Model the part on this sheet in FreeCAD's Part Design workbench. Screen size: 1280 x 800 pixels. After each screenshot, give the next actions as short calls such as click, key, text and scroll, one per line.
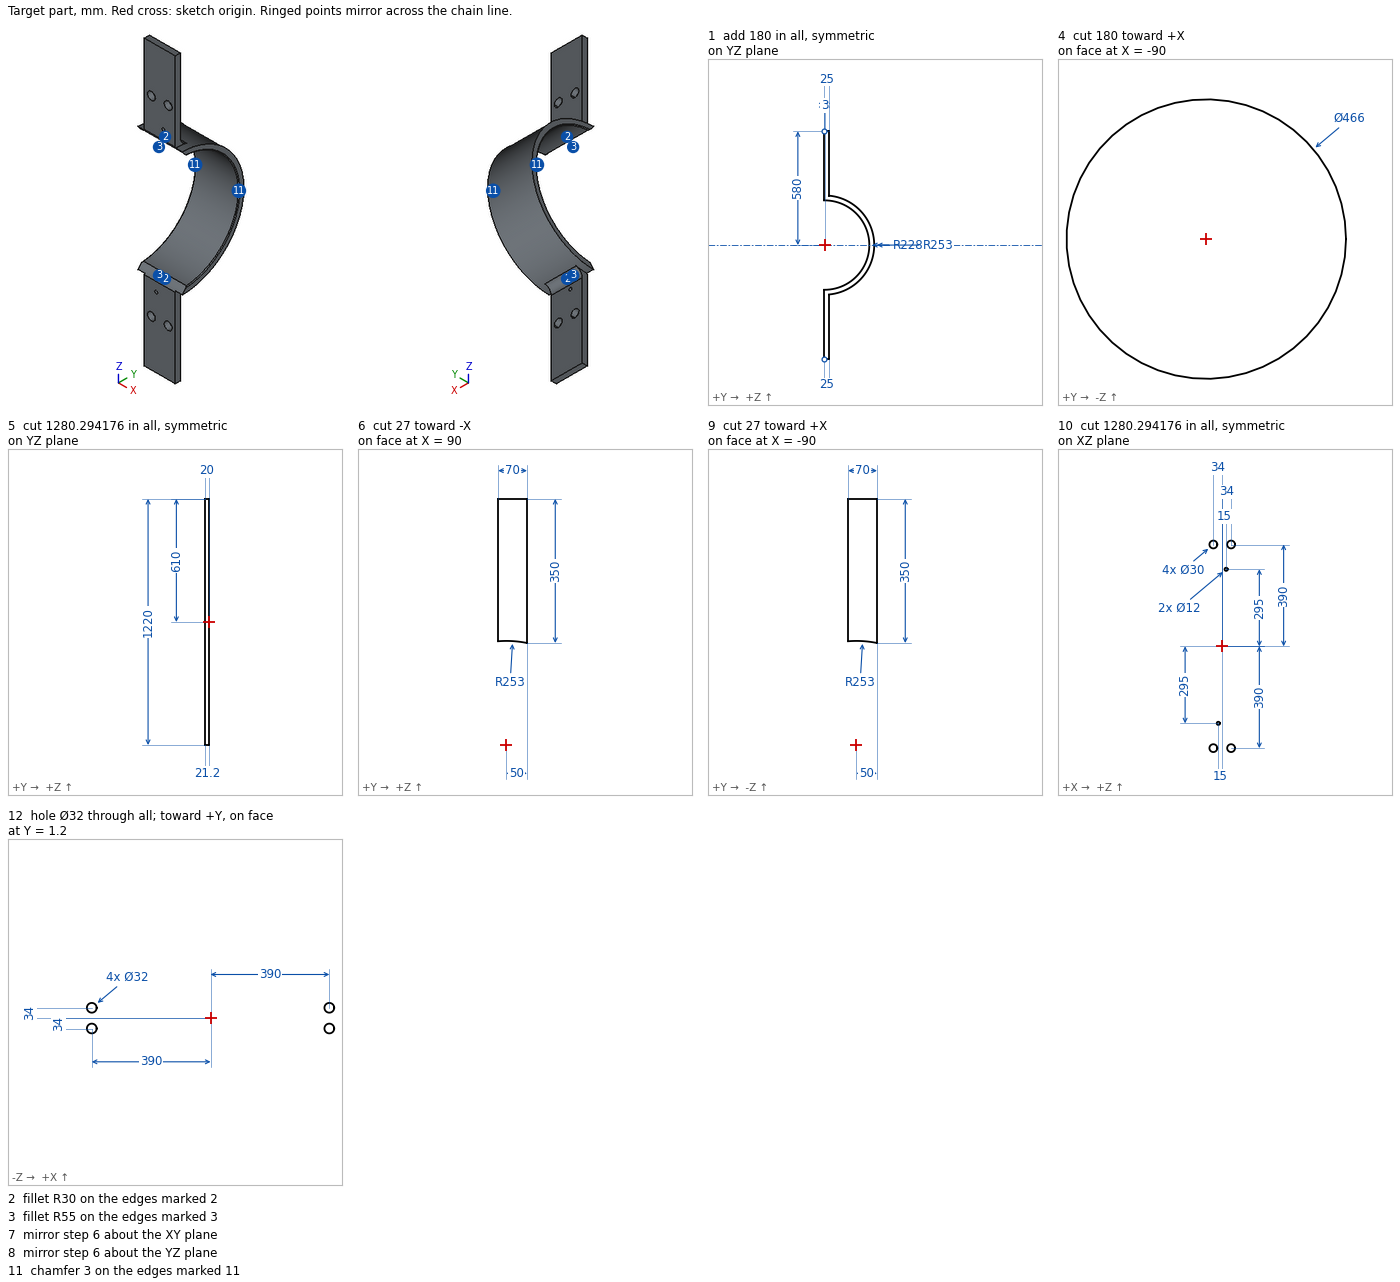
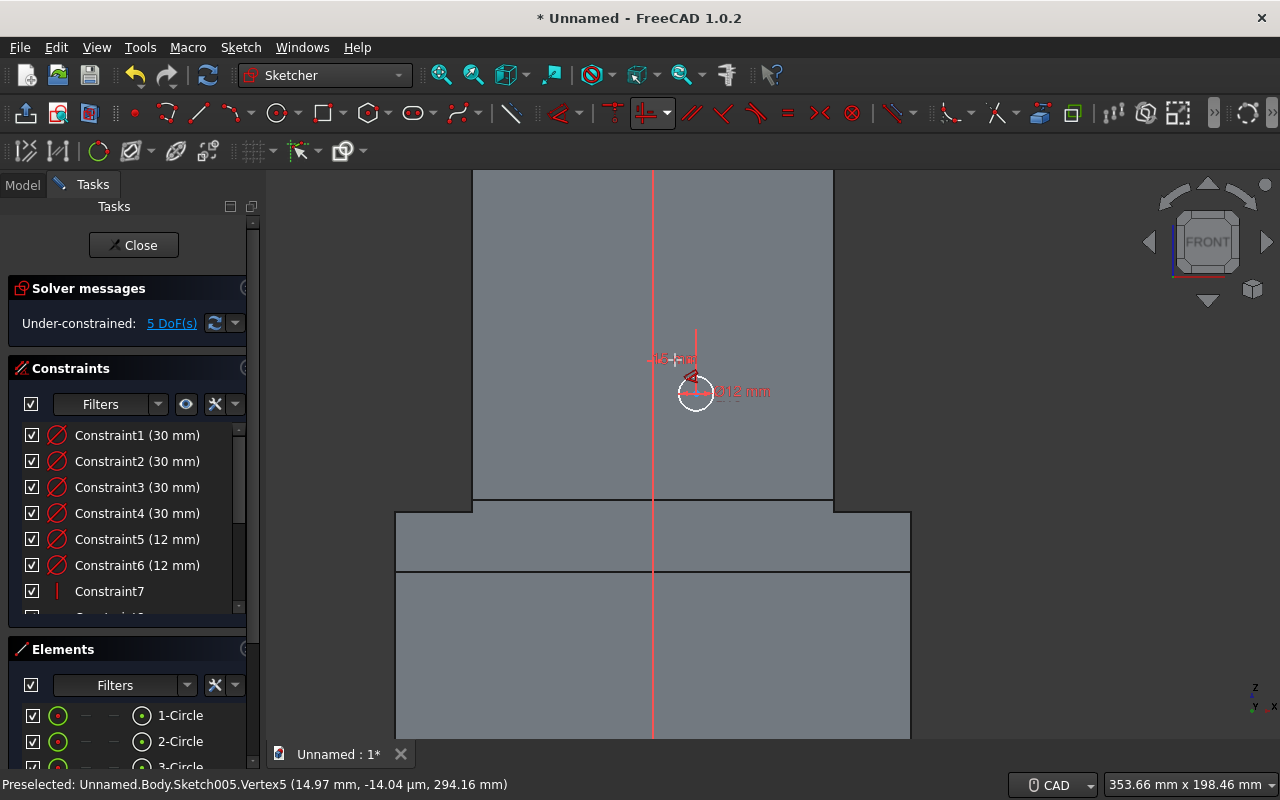
scroll(715, 300, down, 9)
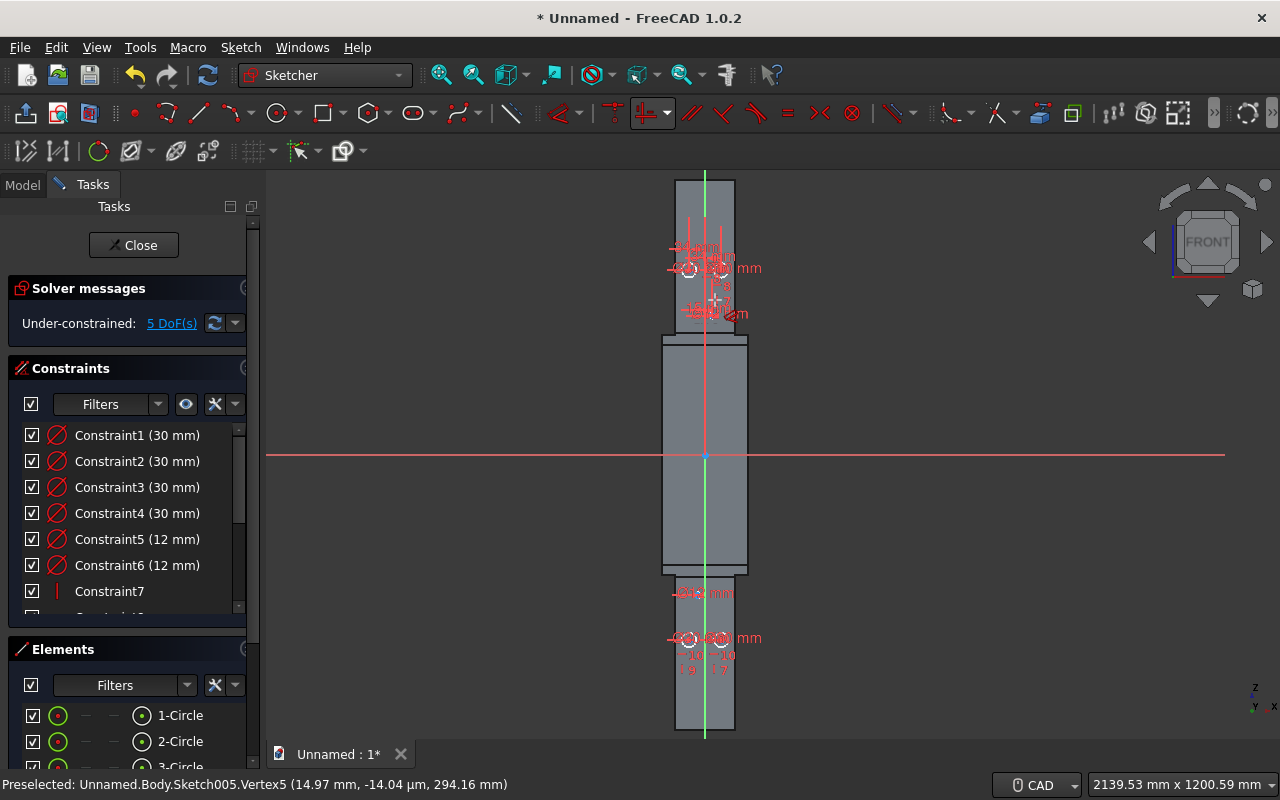
scroll(698, 595, up, 9)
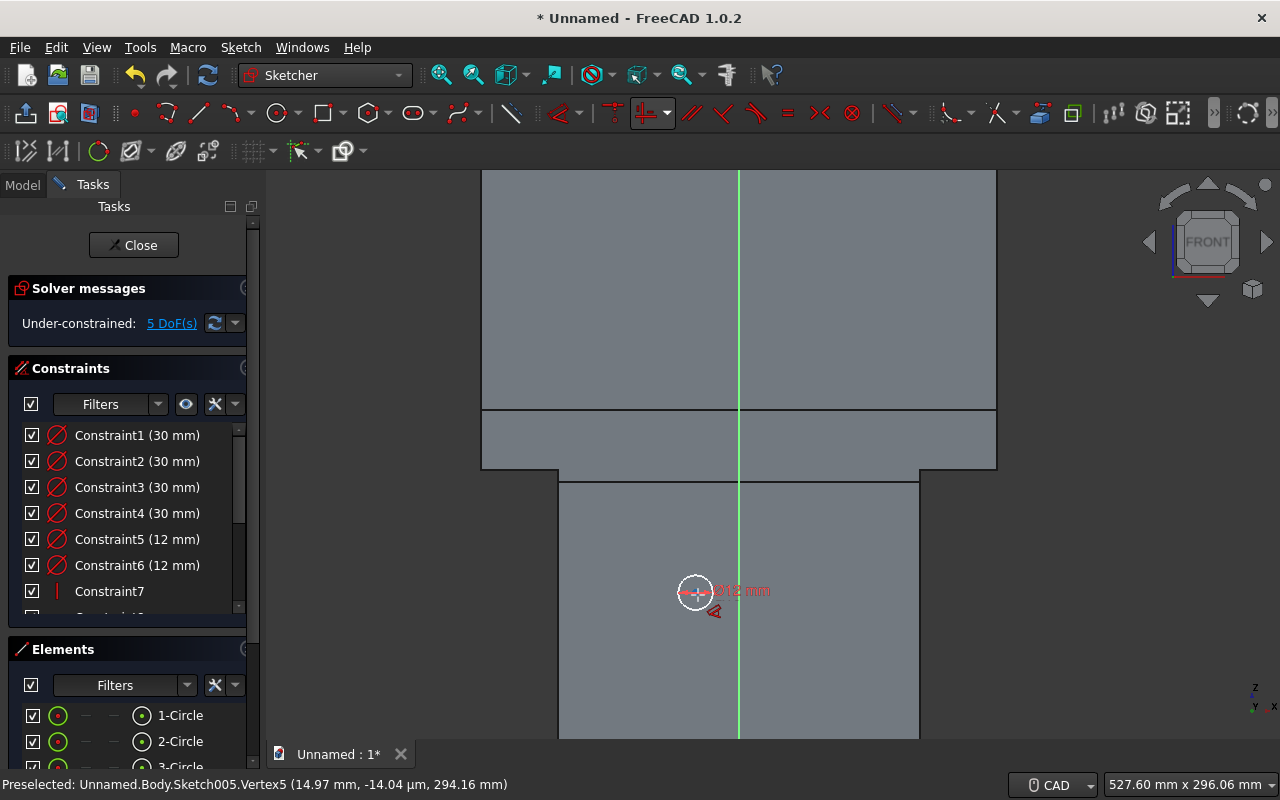
click(696, 593)
click(717, 627)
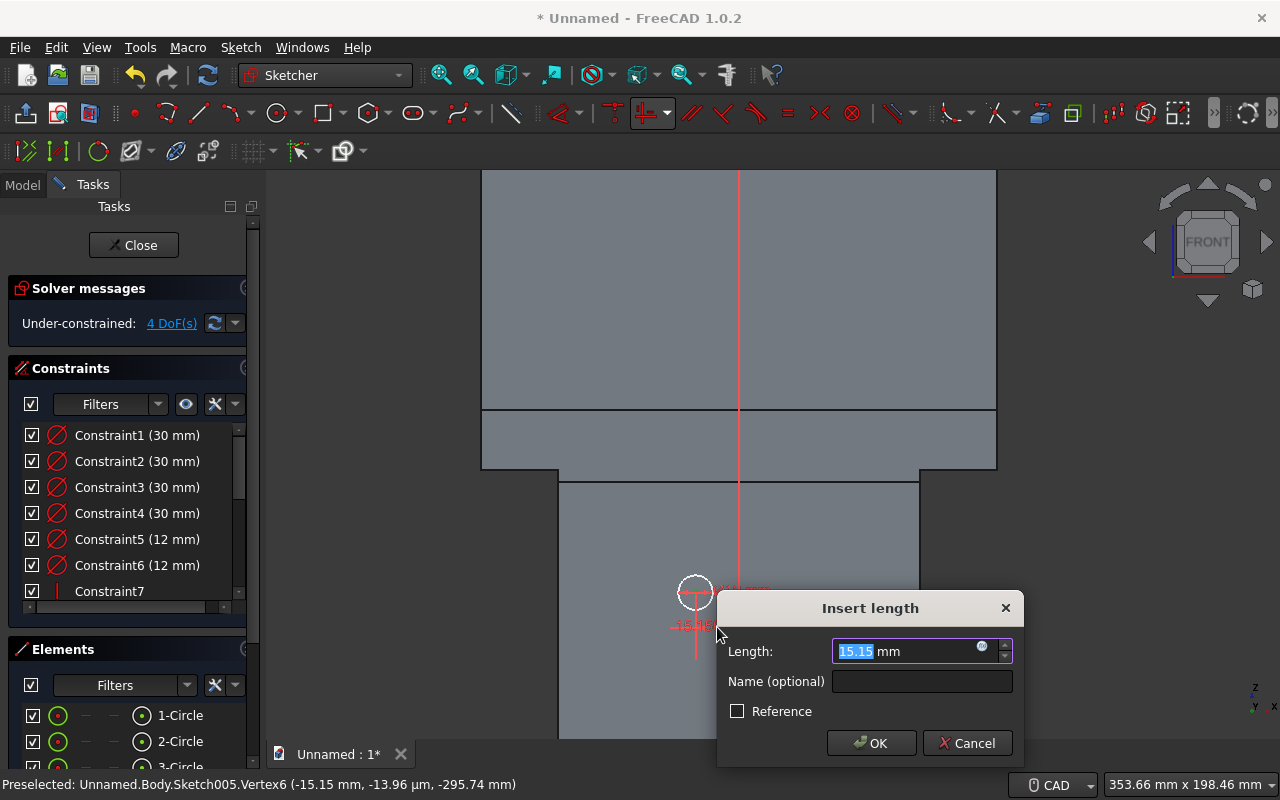
text(15)
key(Return)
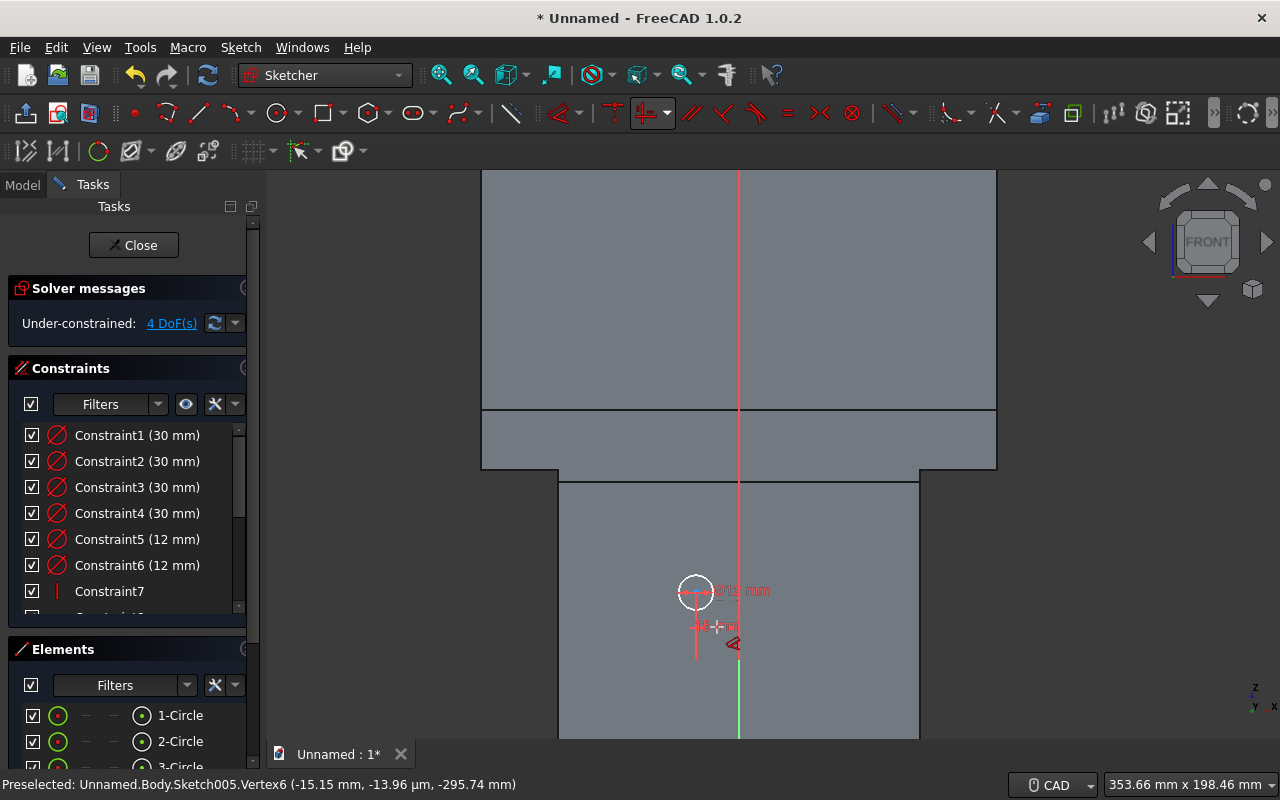
scroll(698, 595, down, 9)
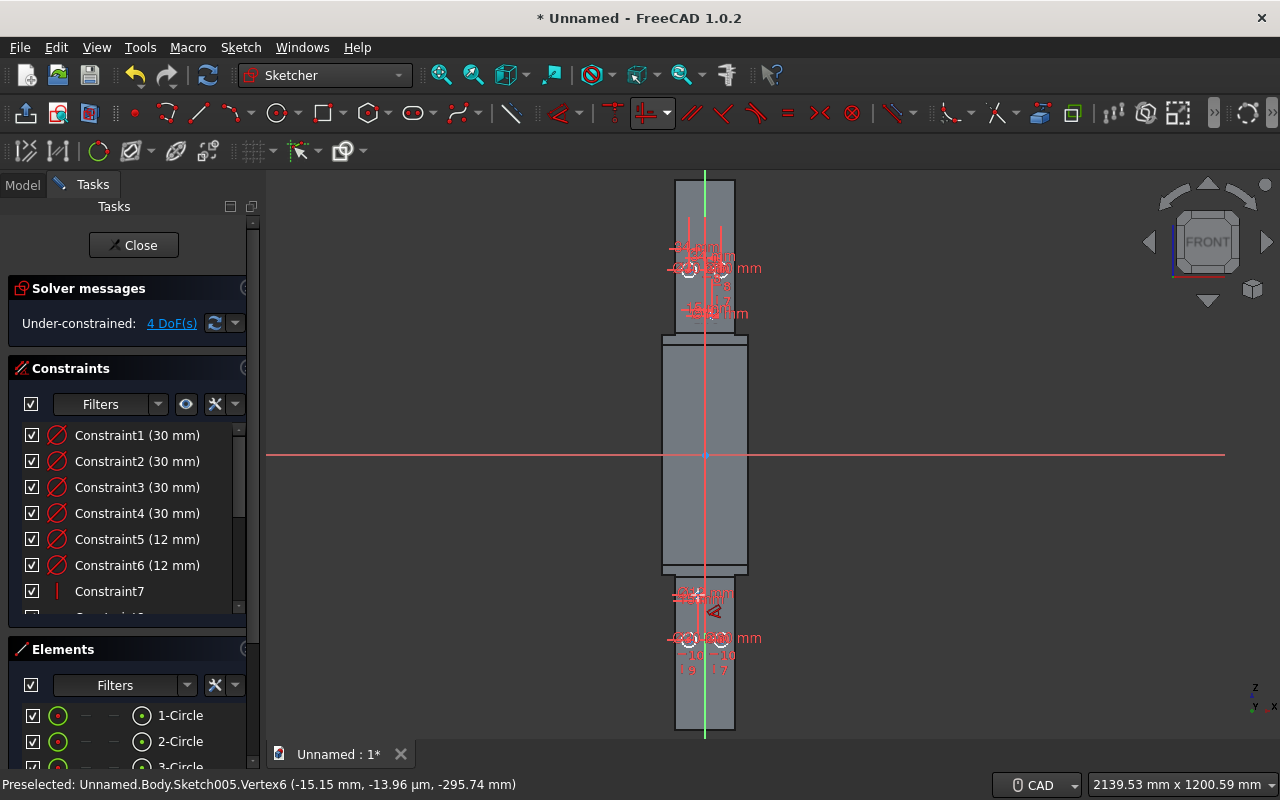
click(721, 270)
click(755, 363)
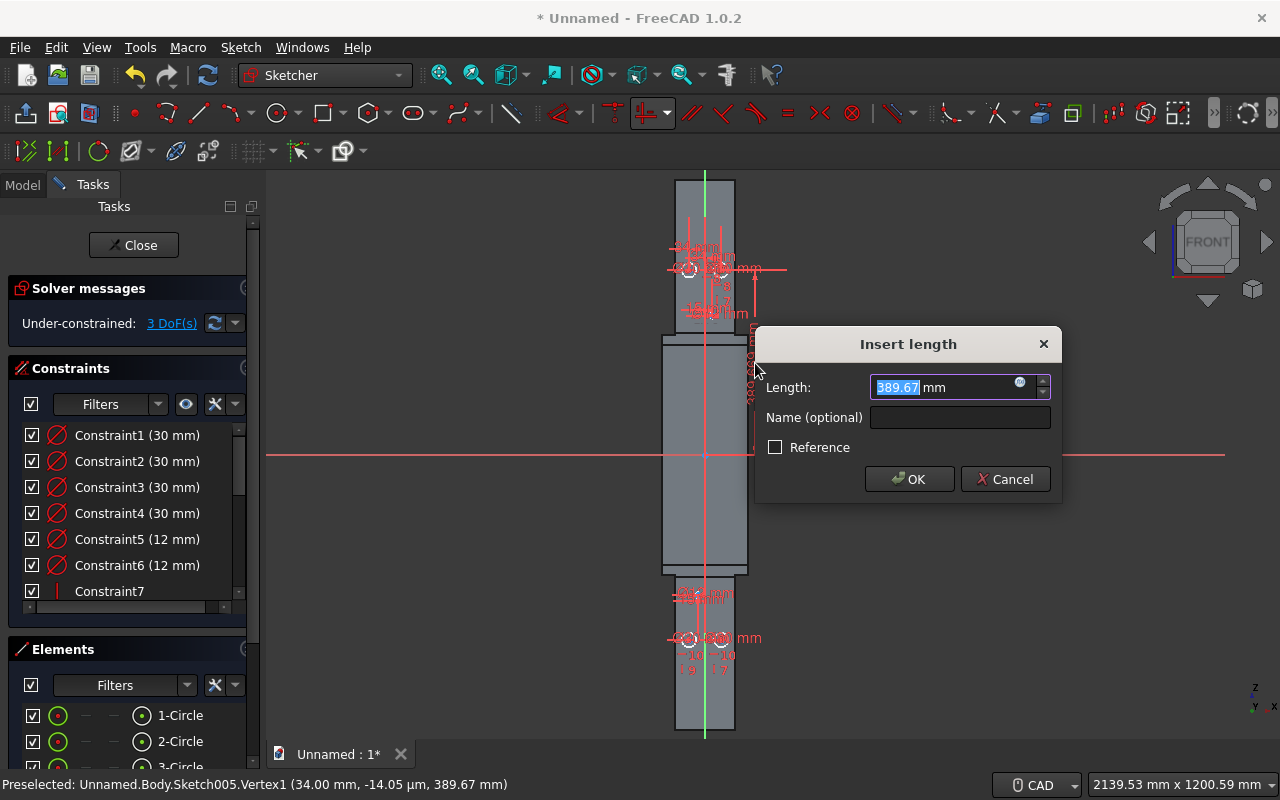
text(390)
key(Return)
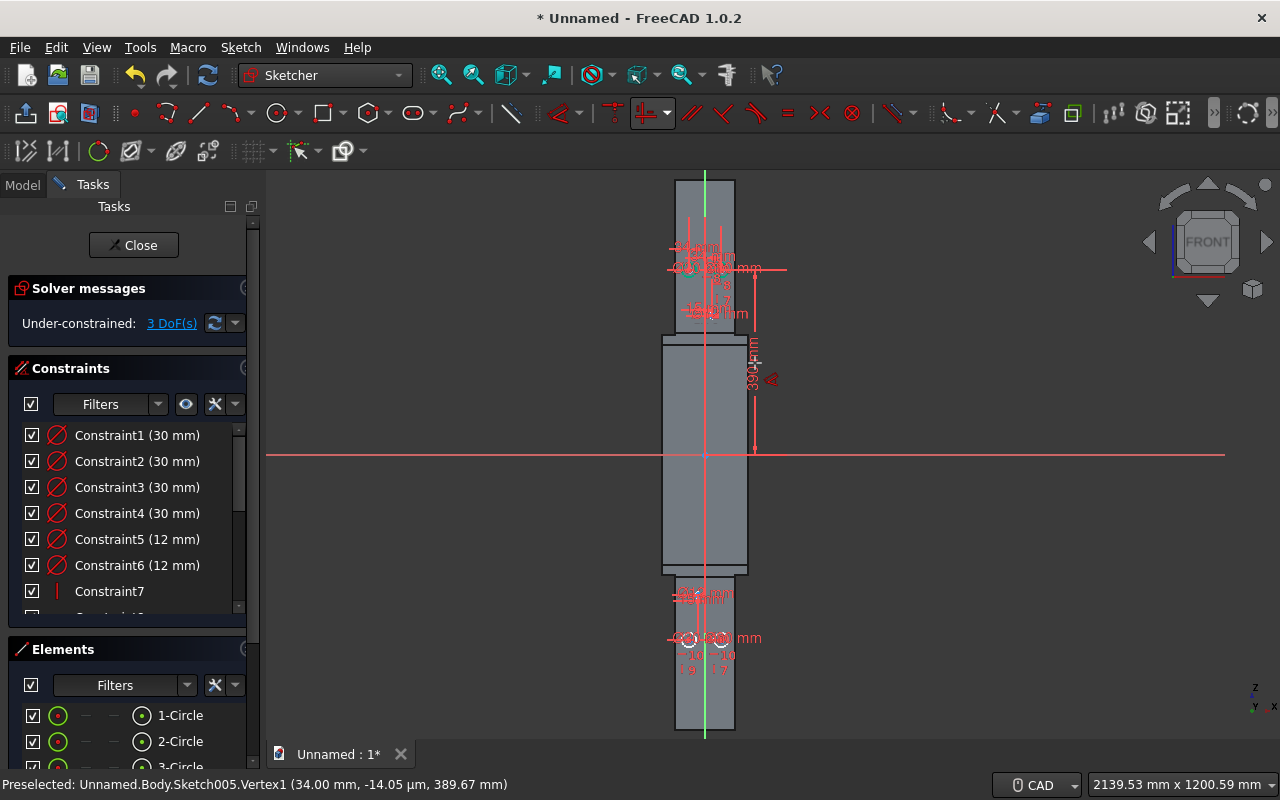
click(721, 640)
click(755, 548)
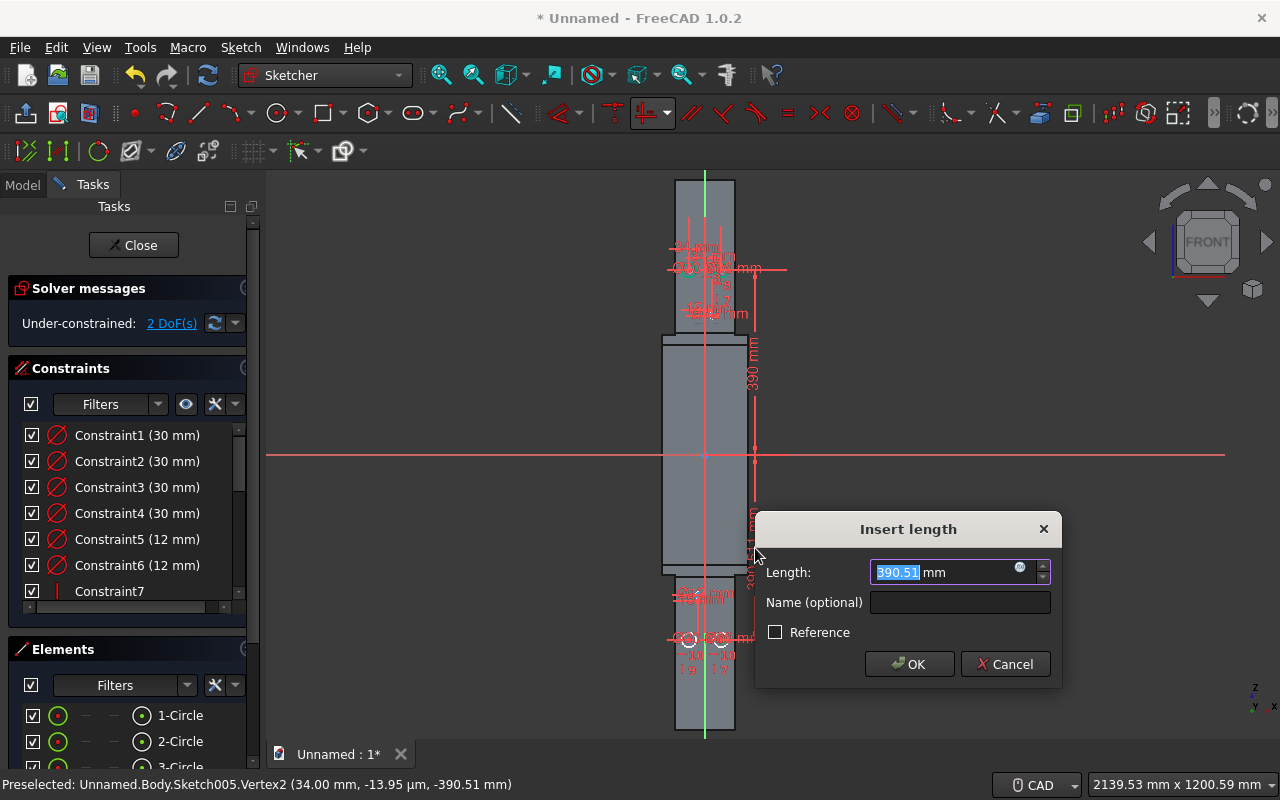
text(390)
key(Return)